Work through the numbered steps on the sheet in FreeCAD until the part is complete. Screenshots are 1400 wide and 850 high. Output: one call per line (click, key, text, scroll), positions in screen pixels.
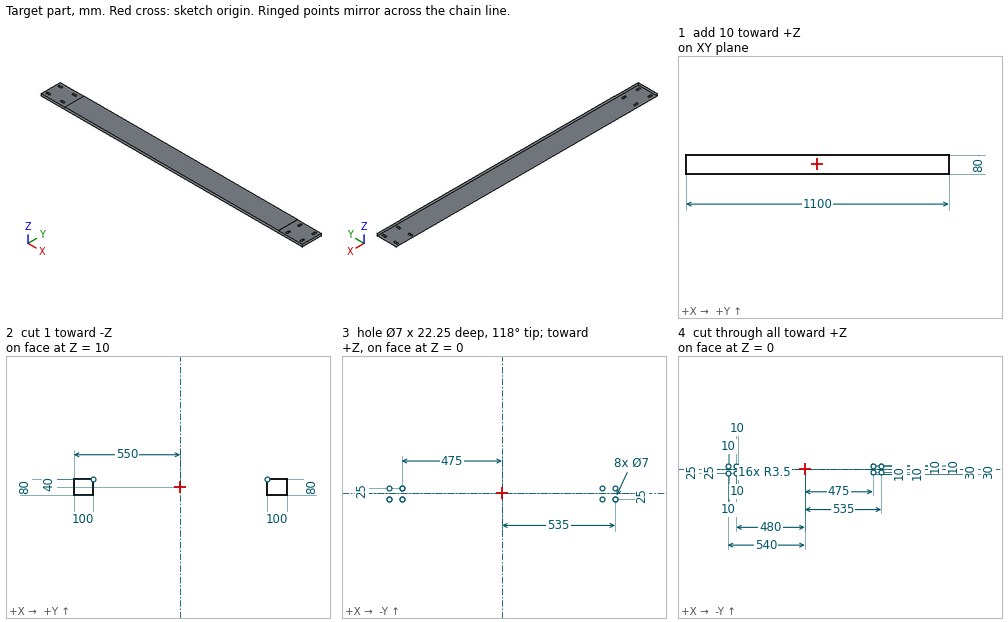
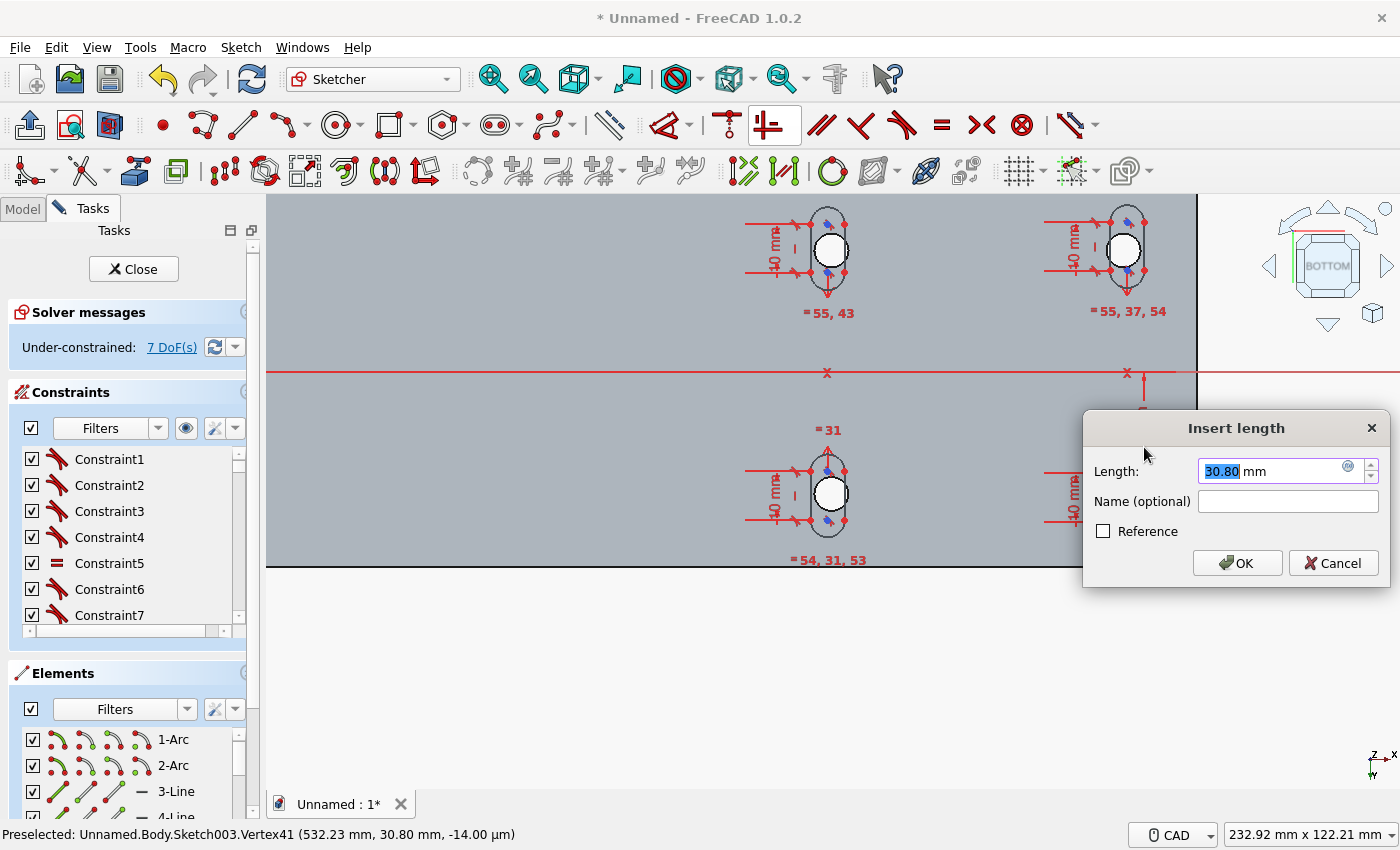
text(30)
key(Return)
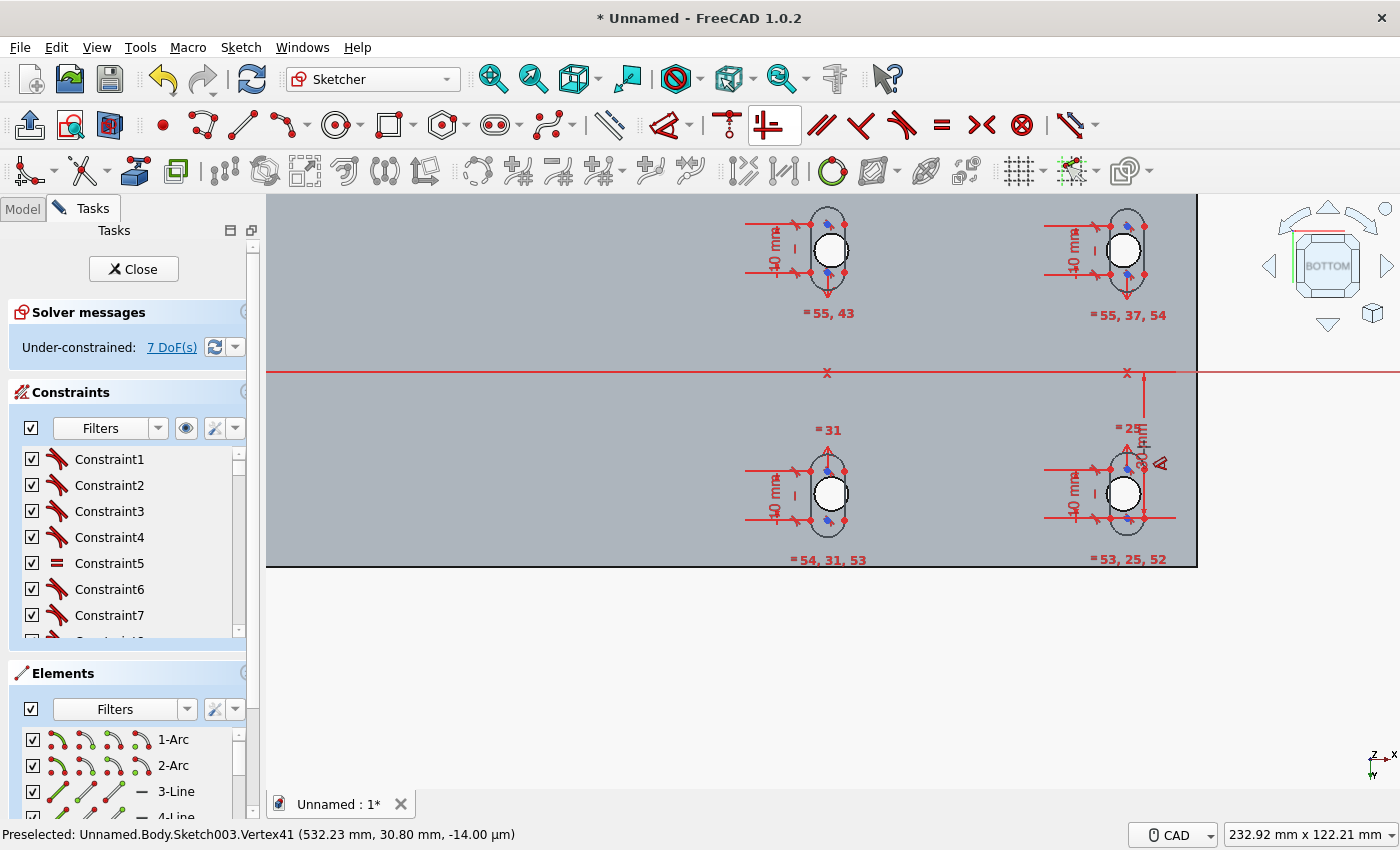
click(811, 520)
click(845, 446)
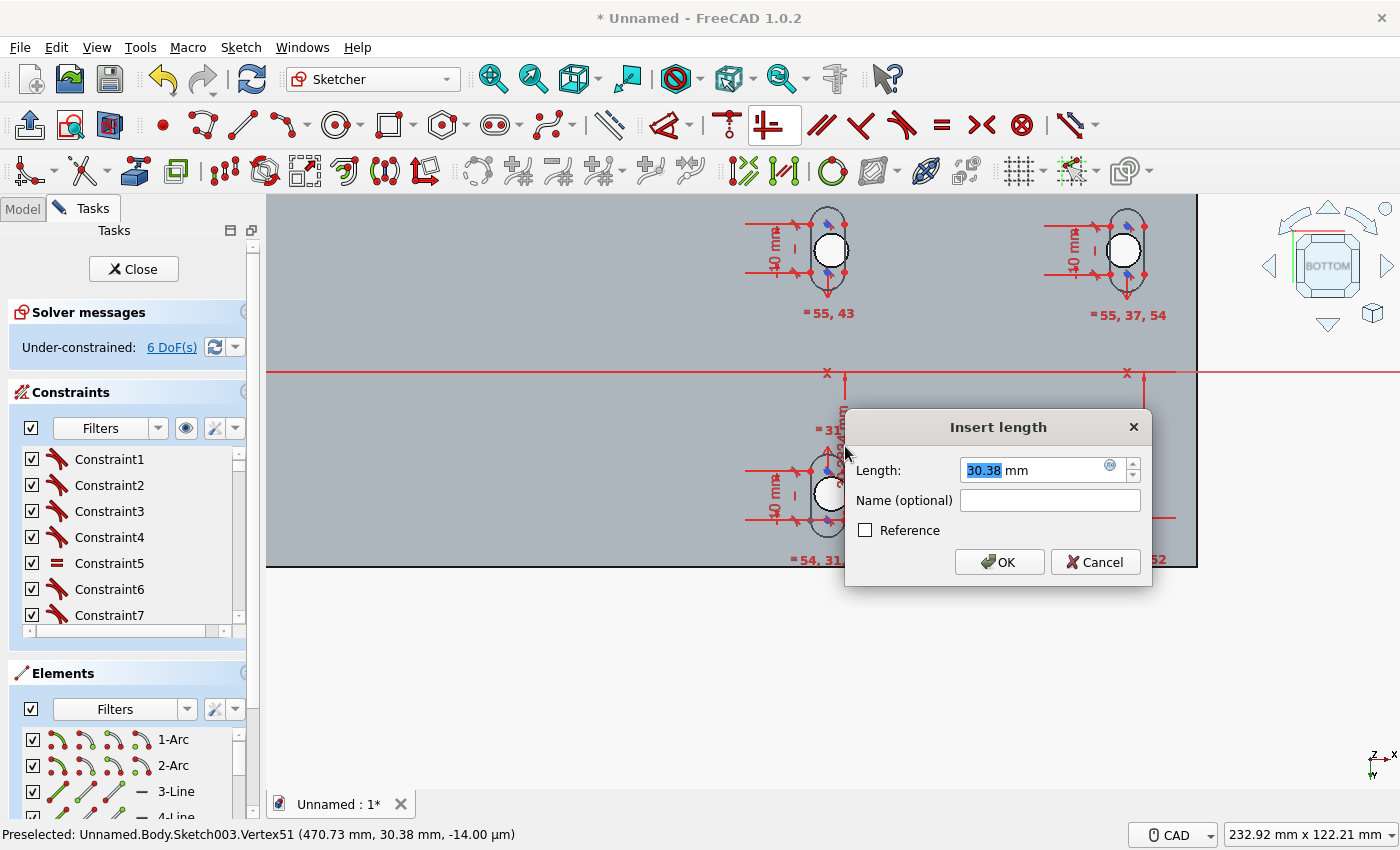
text(30)
key(Return)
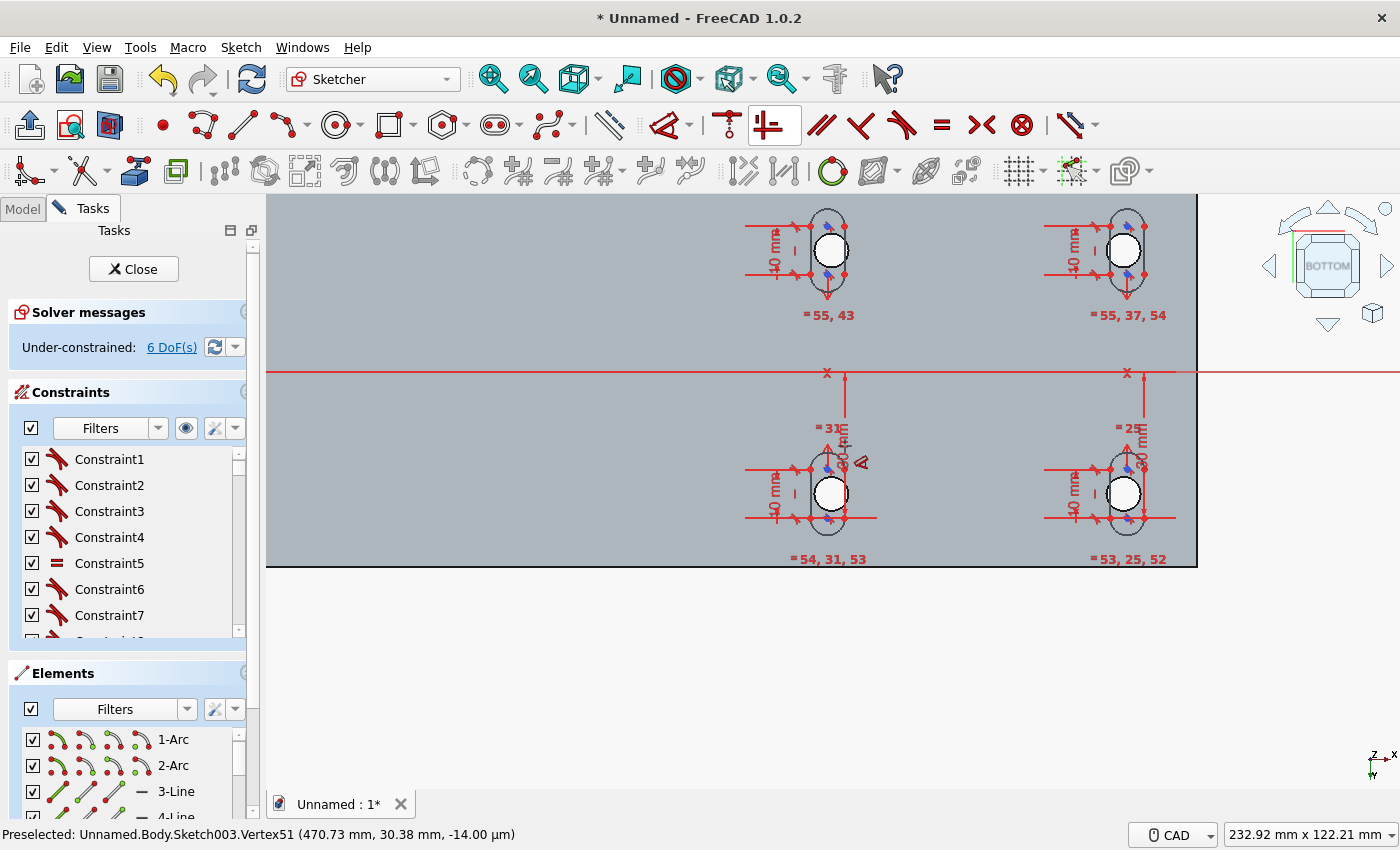
scroll(1118, 510, down, 10)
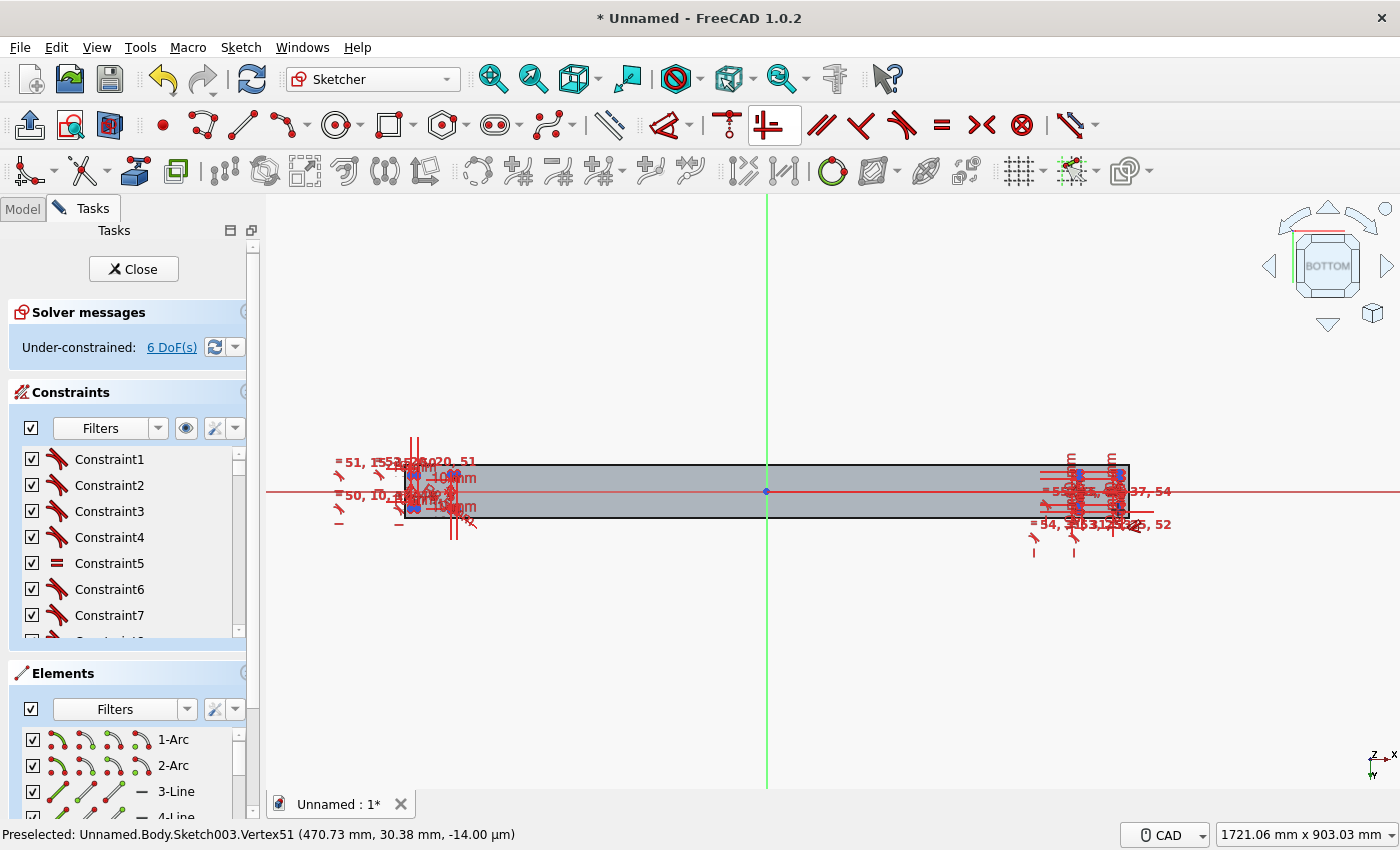
scroll(451, 509, up, 9)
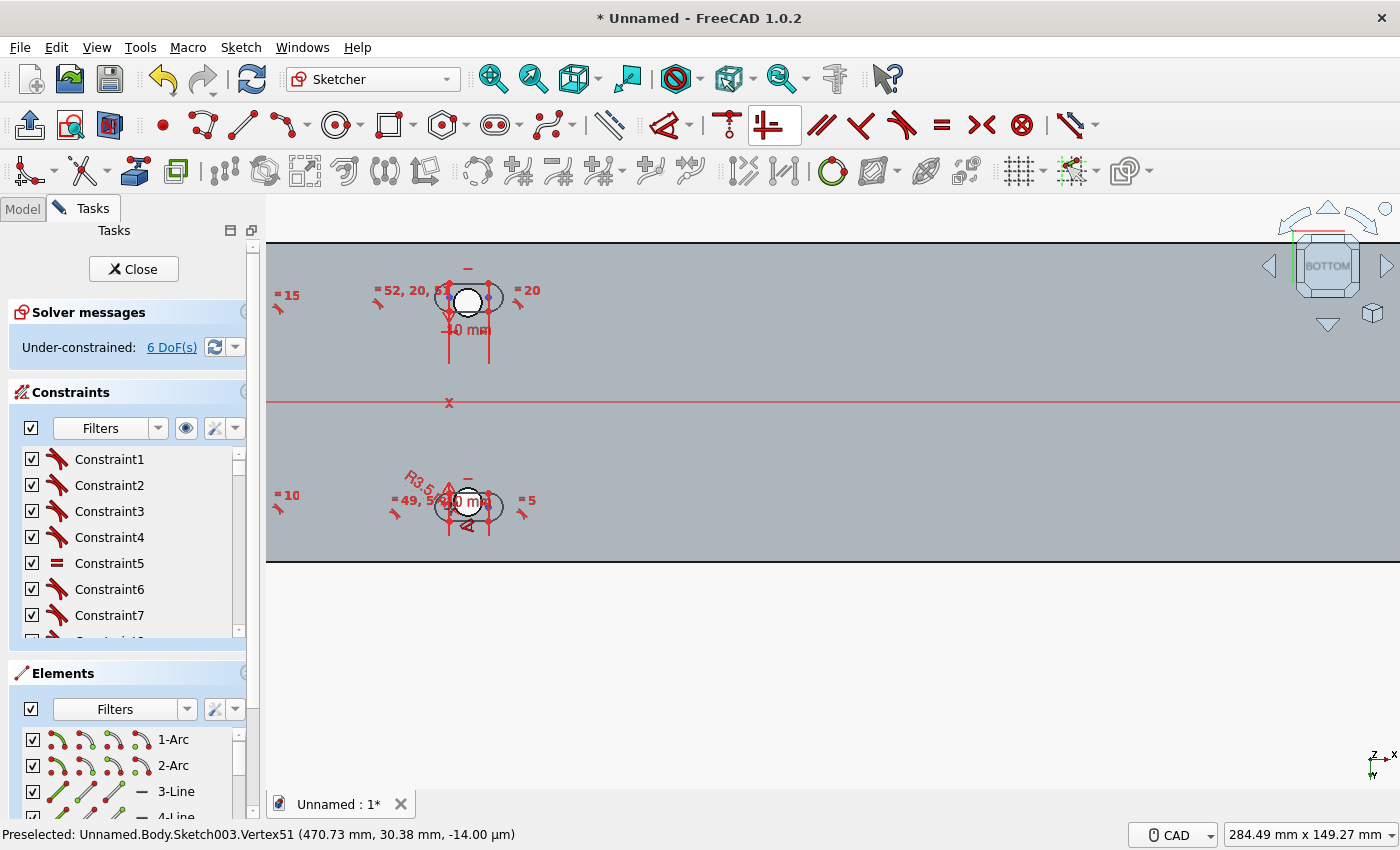
click(449, 507)
click(415, 455)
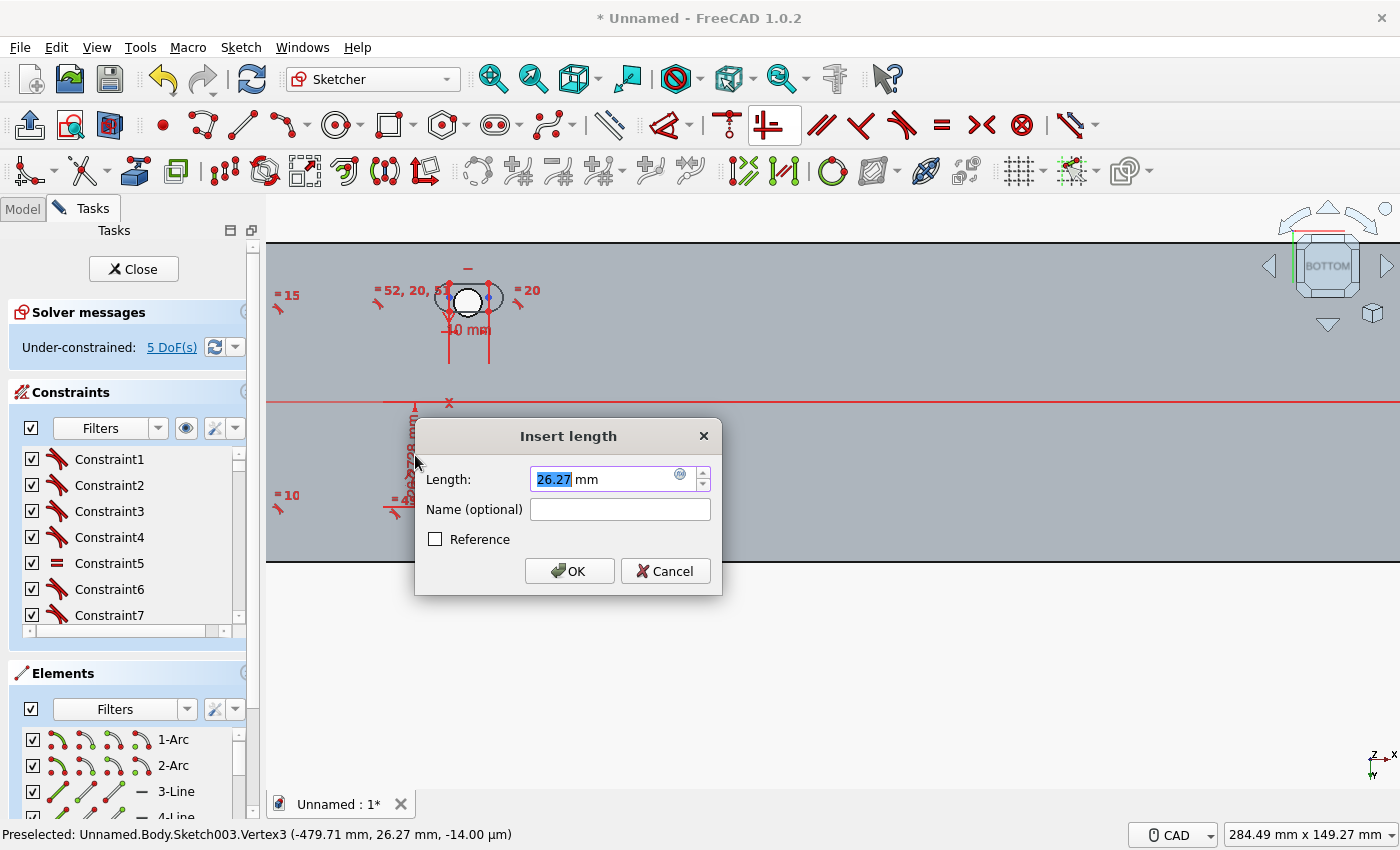
text(25)
key(Return)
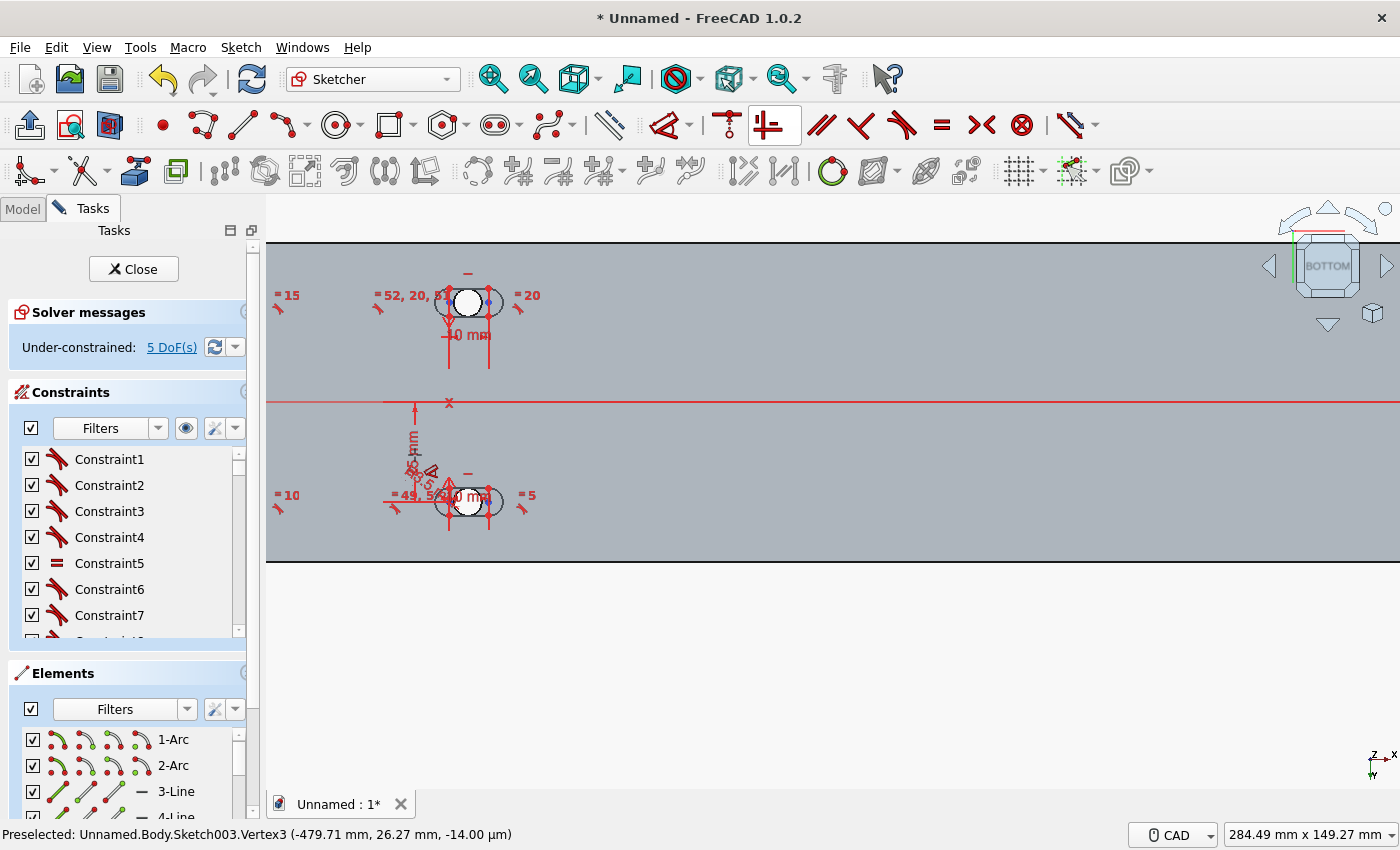
scroll(450, 509, down, 9)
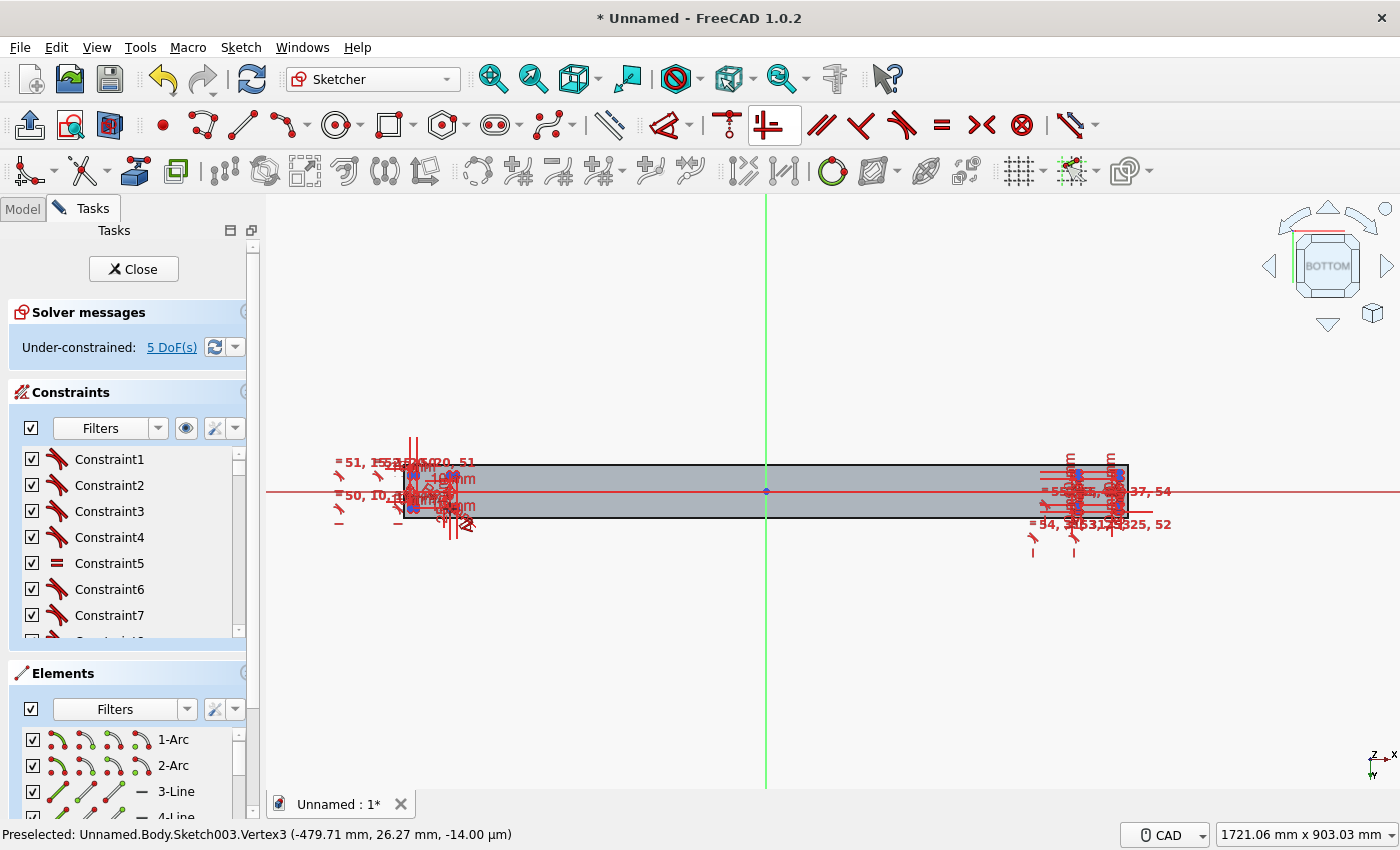
scroll(410, 508, up, 9)